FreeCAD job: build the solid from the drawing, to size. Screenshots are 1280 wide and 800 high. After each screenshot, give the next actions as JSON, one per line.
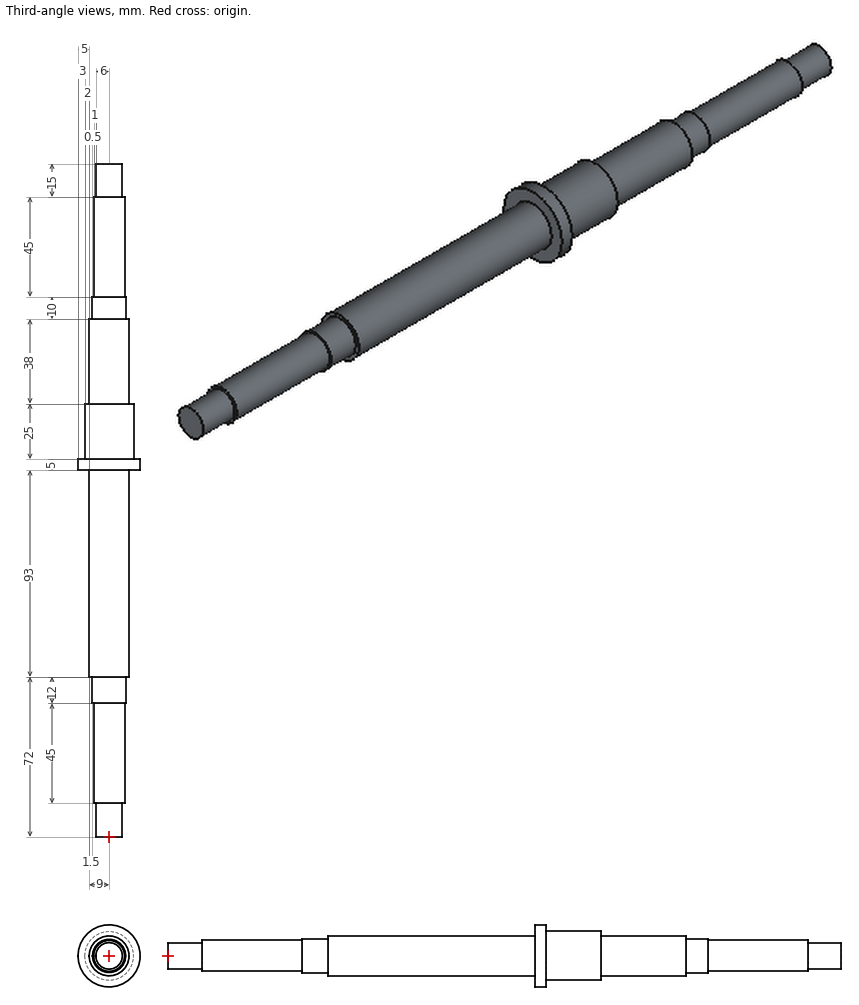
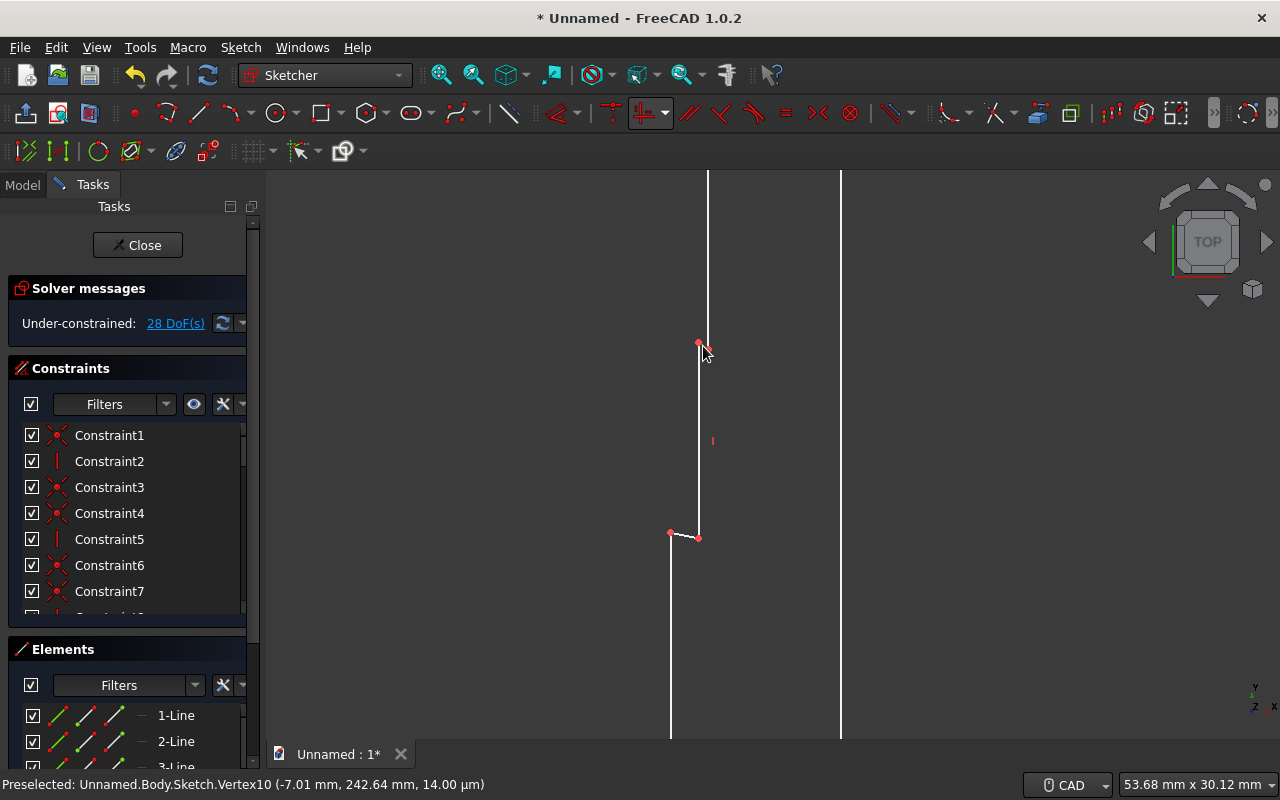
{"action": "key", "text": "h"}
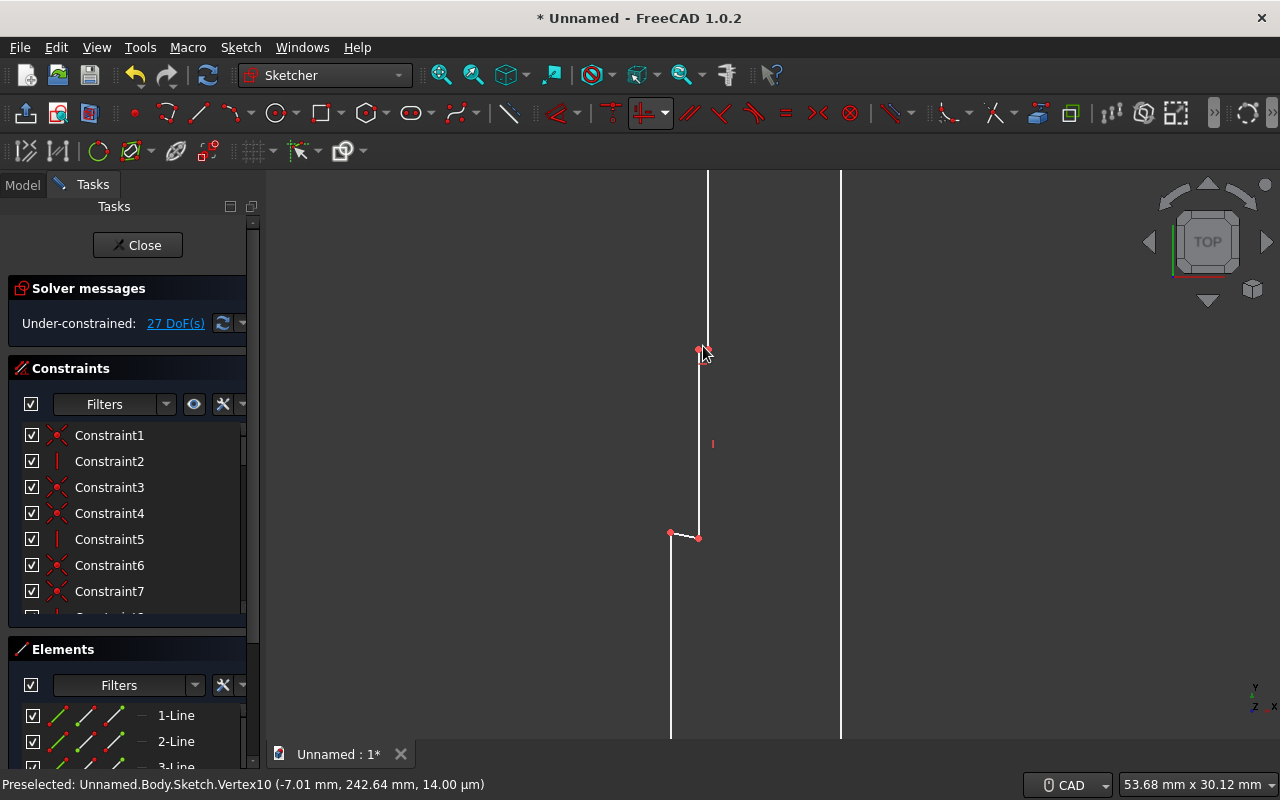
{"action": "left_click", "coordinate": [688, 536]}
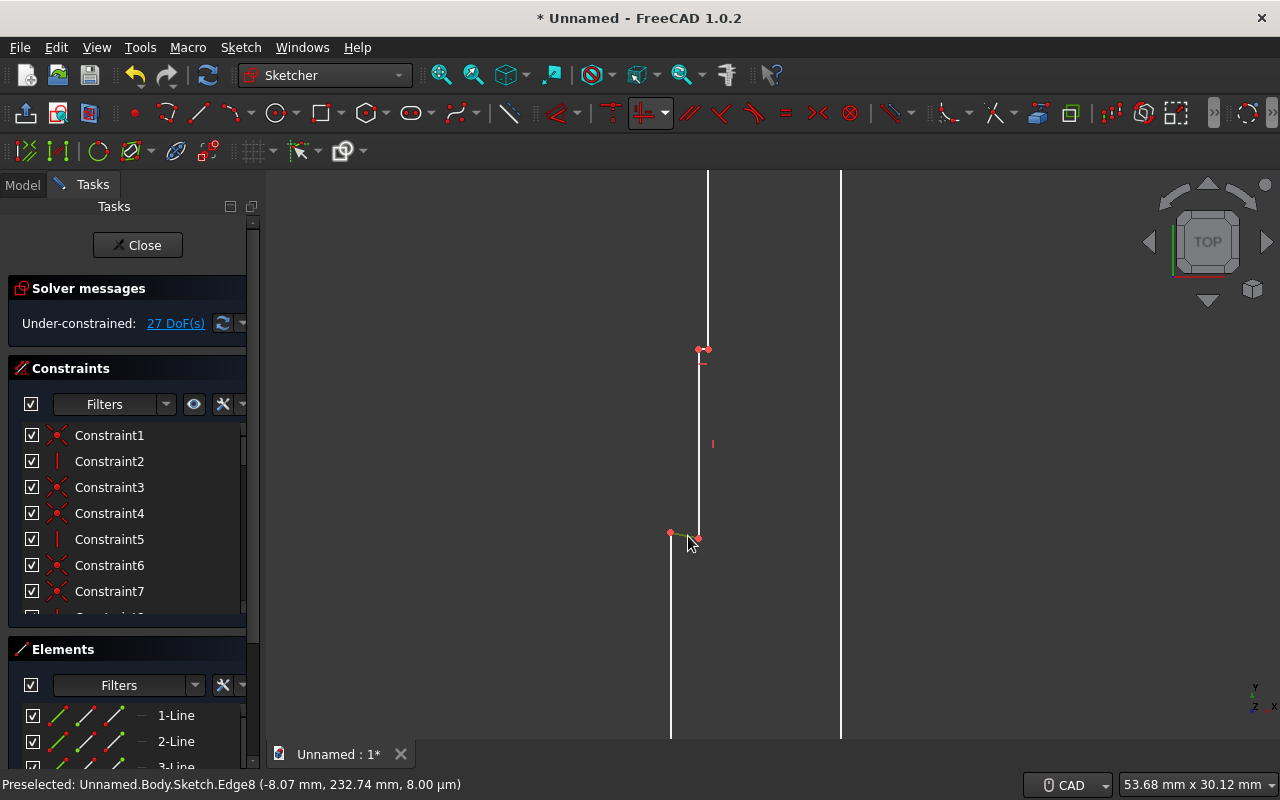
{"action": "key", "text": "h"}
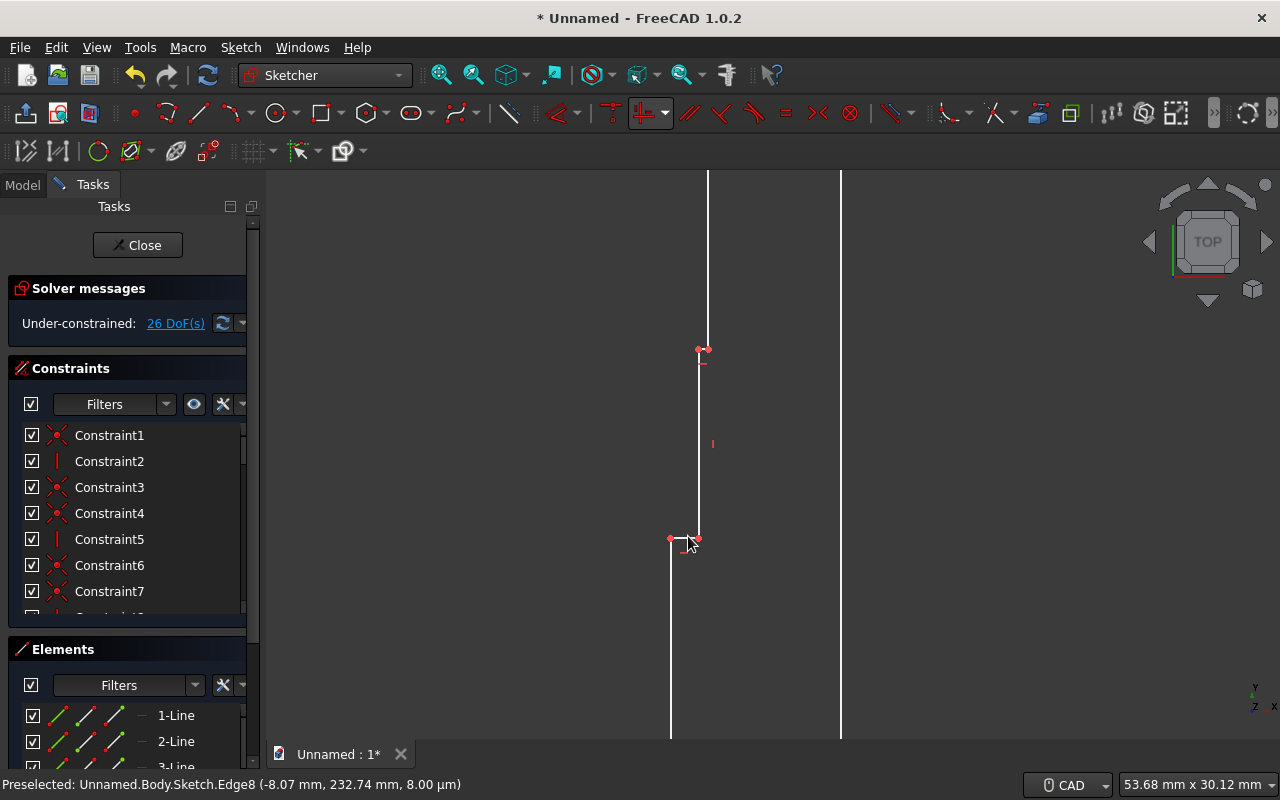
{"action": "scroll", "coordinate": [704, 350], "scroll_direction": "down", "scroll_amount": 14}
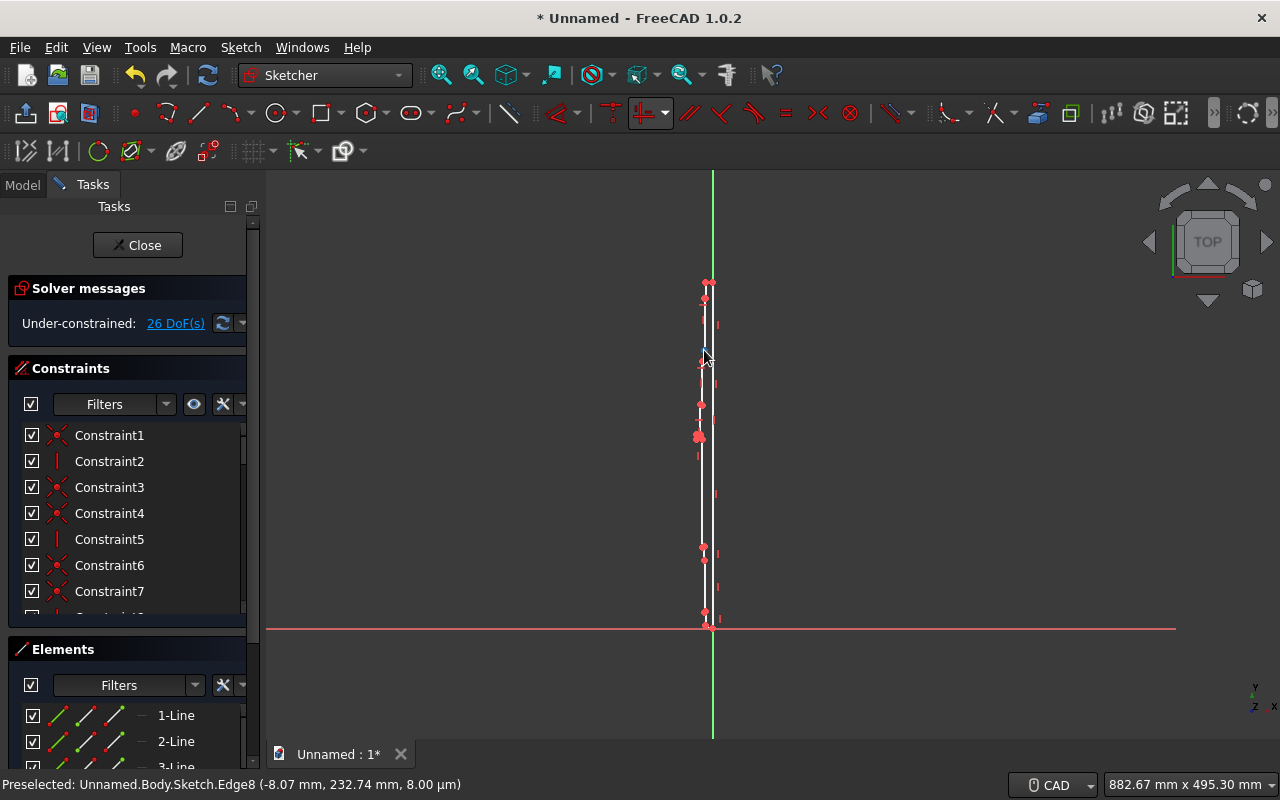
{"action": "scroll", "coordinate": [702, 405], "scroll_direction": "up", "scroll_amount": 14}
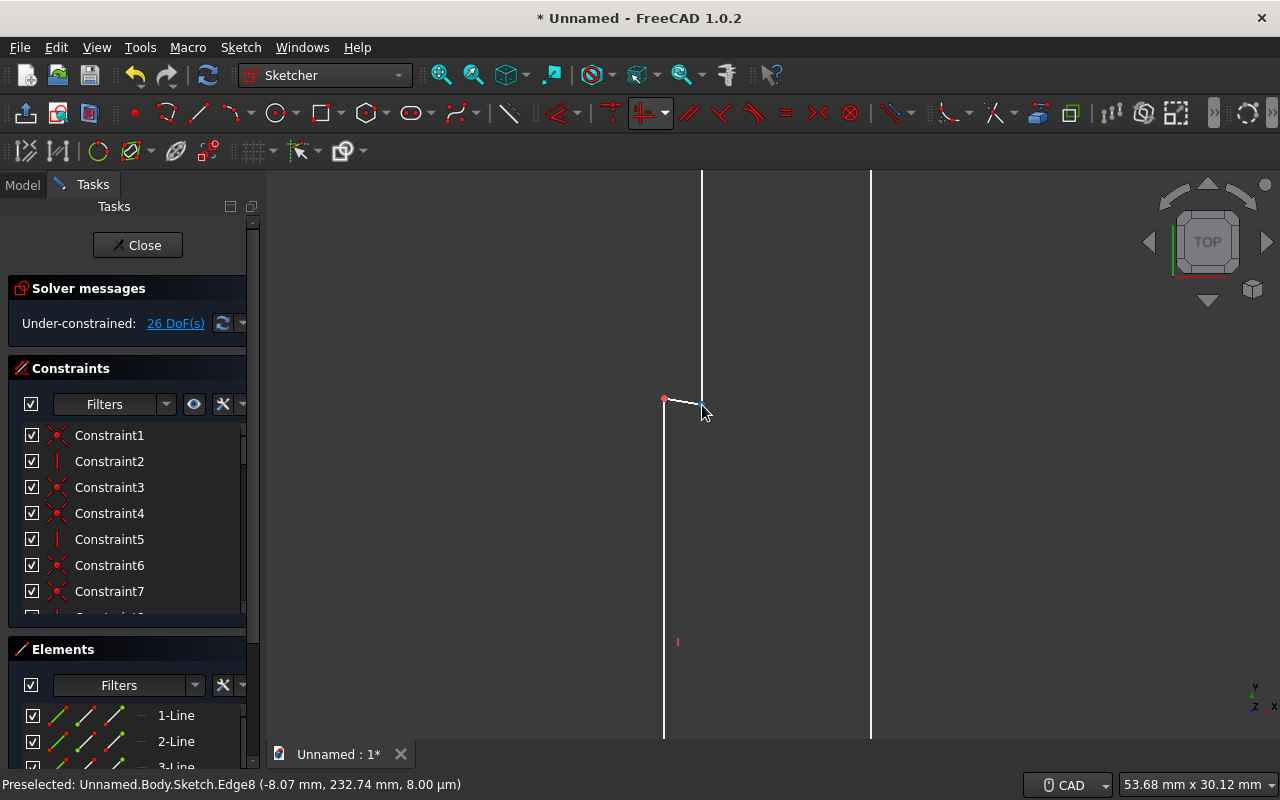
{"action": "left_click", "coordinate": [690, 403]}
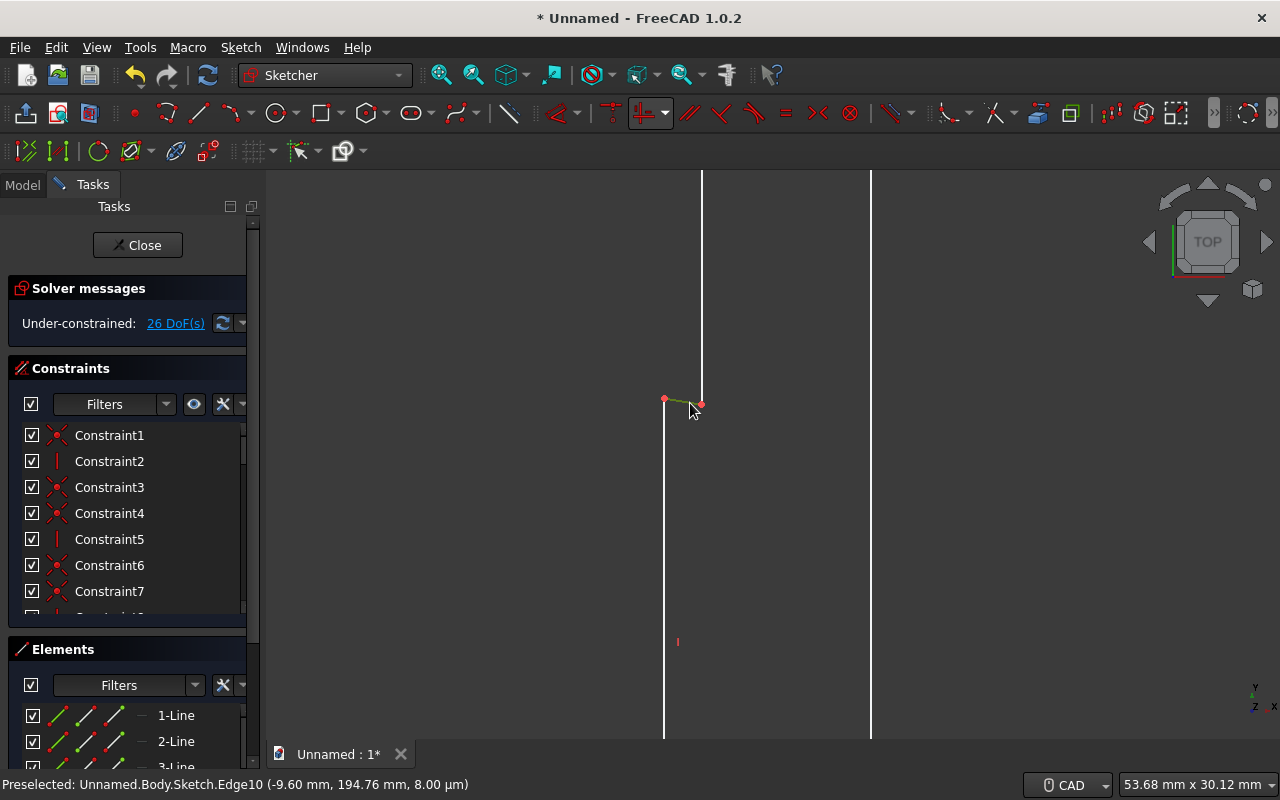
{"action": "key", "text": "h"}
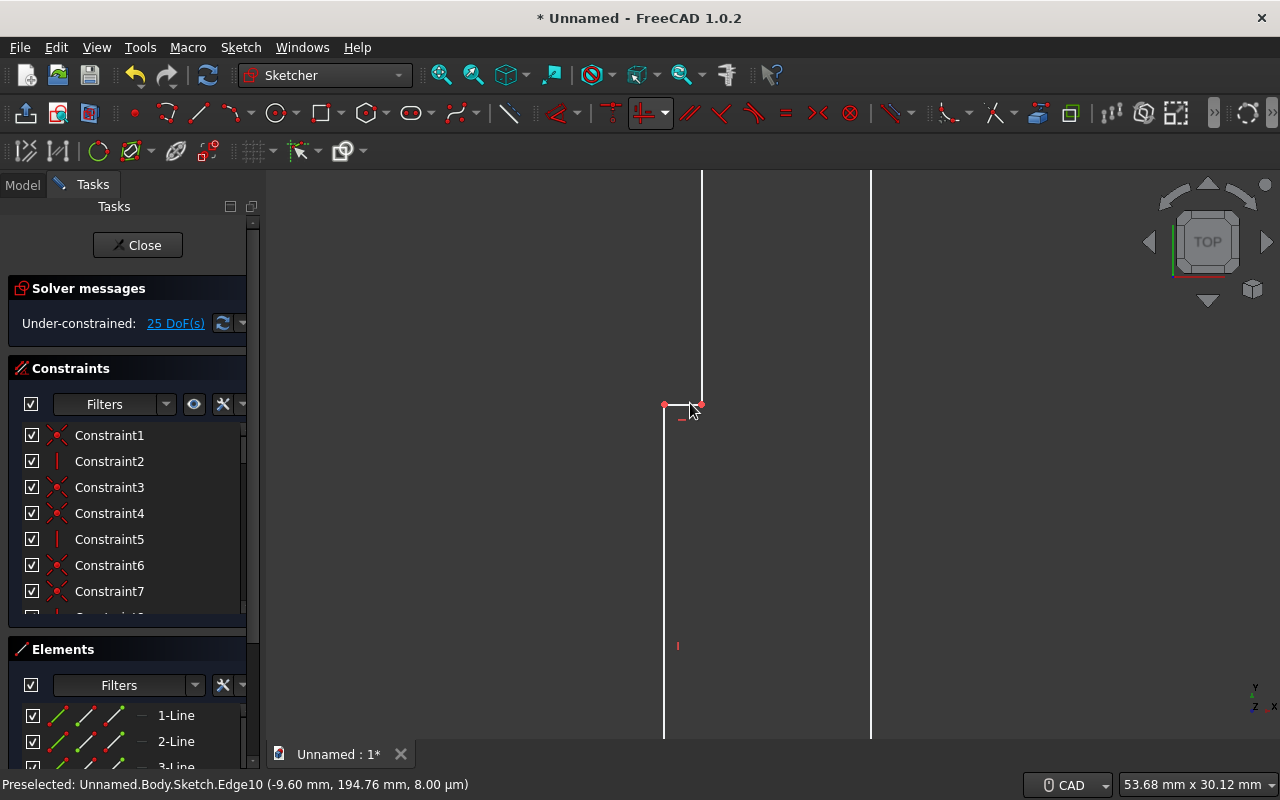
{"action": "scroll", "coordinate": [702, 405], "scroll_direction": "down", "scroll_amount": 14}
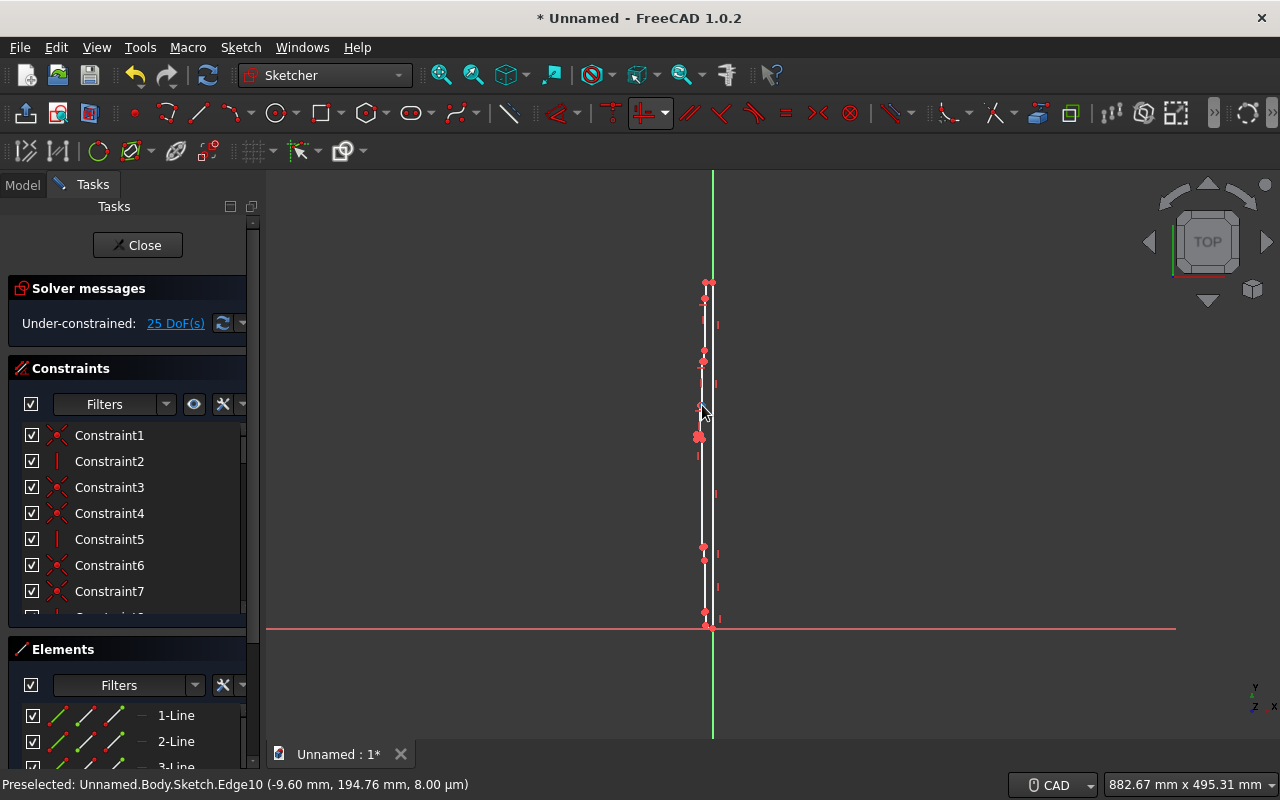
{"action": "scroll", "coordinate": [699, 434], "scroll_direction": "up", "scroll_amount": 13}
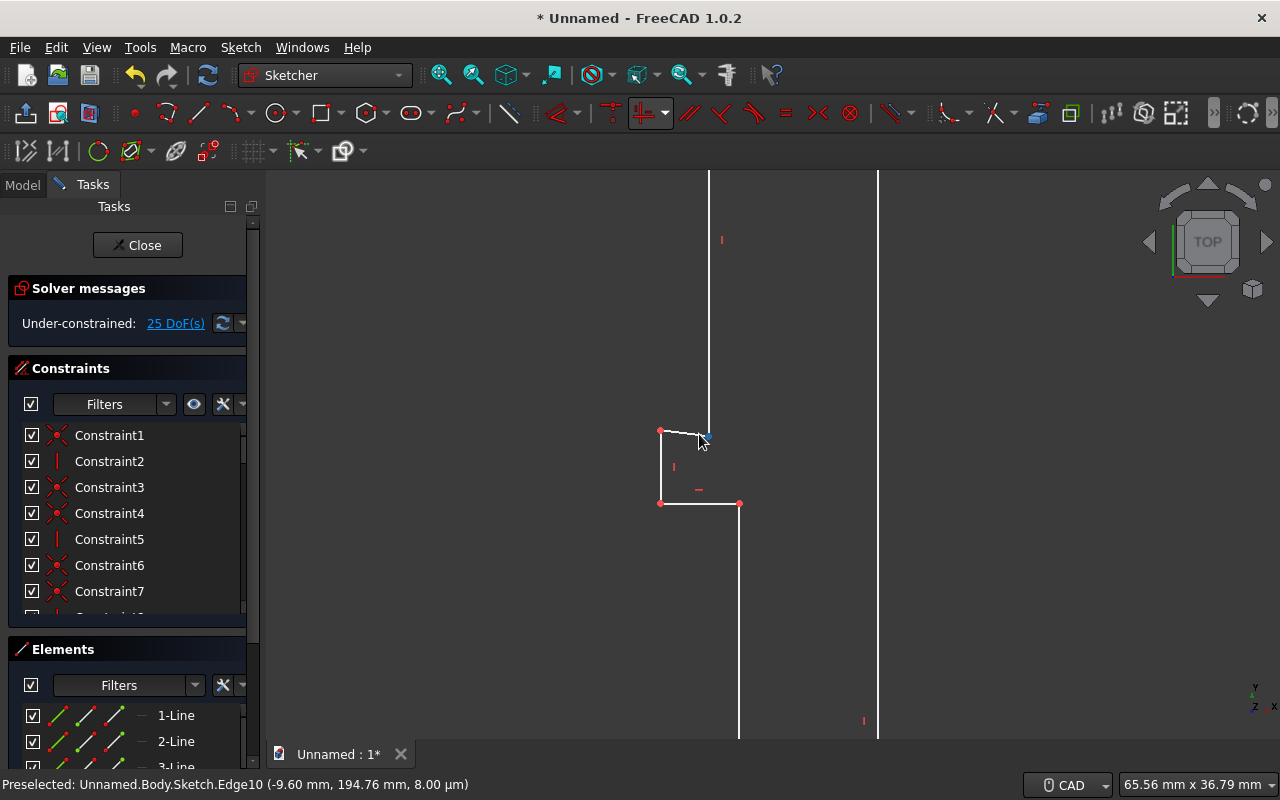
{"action": "left_click", "coordinate": [694, 434]}